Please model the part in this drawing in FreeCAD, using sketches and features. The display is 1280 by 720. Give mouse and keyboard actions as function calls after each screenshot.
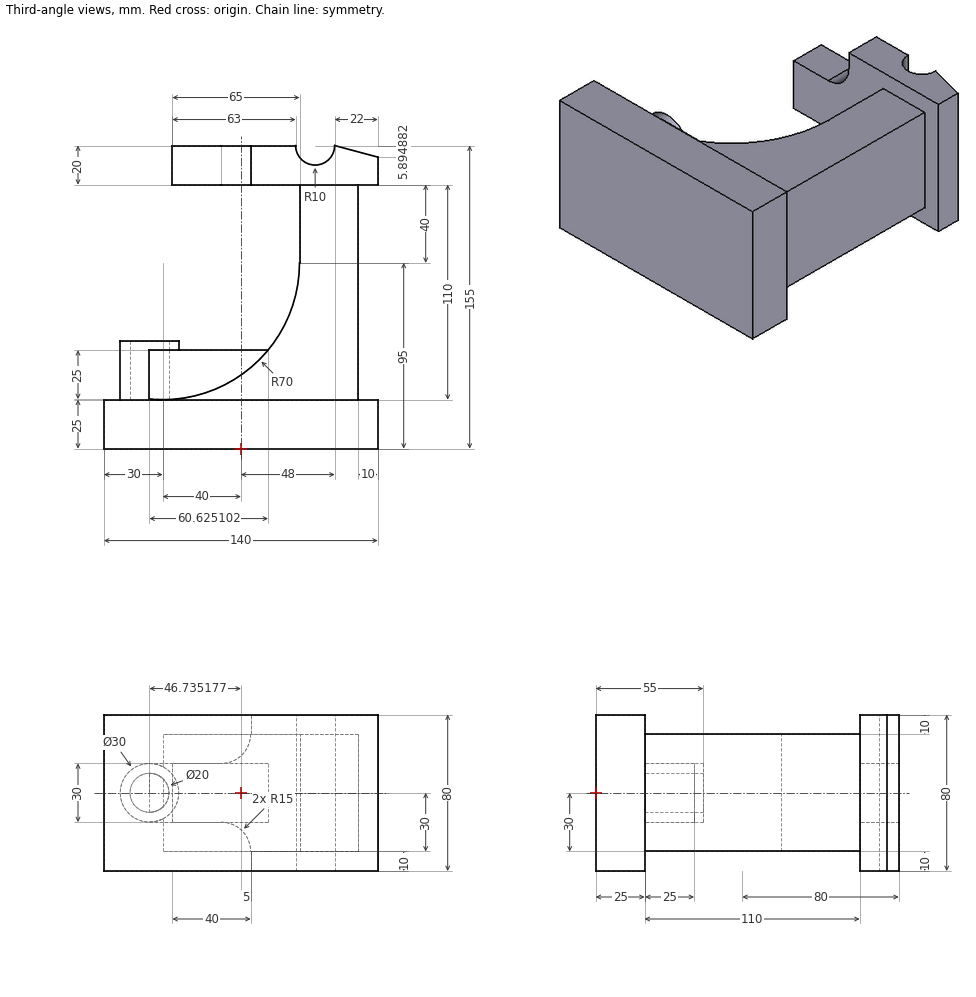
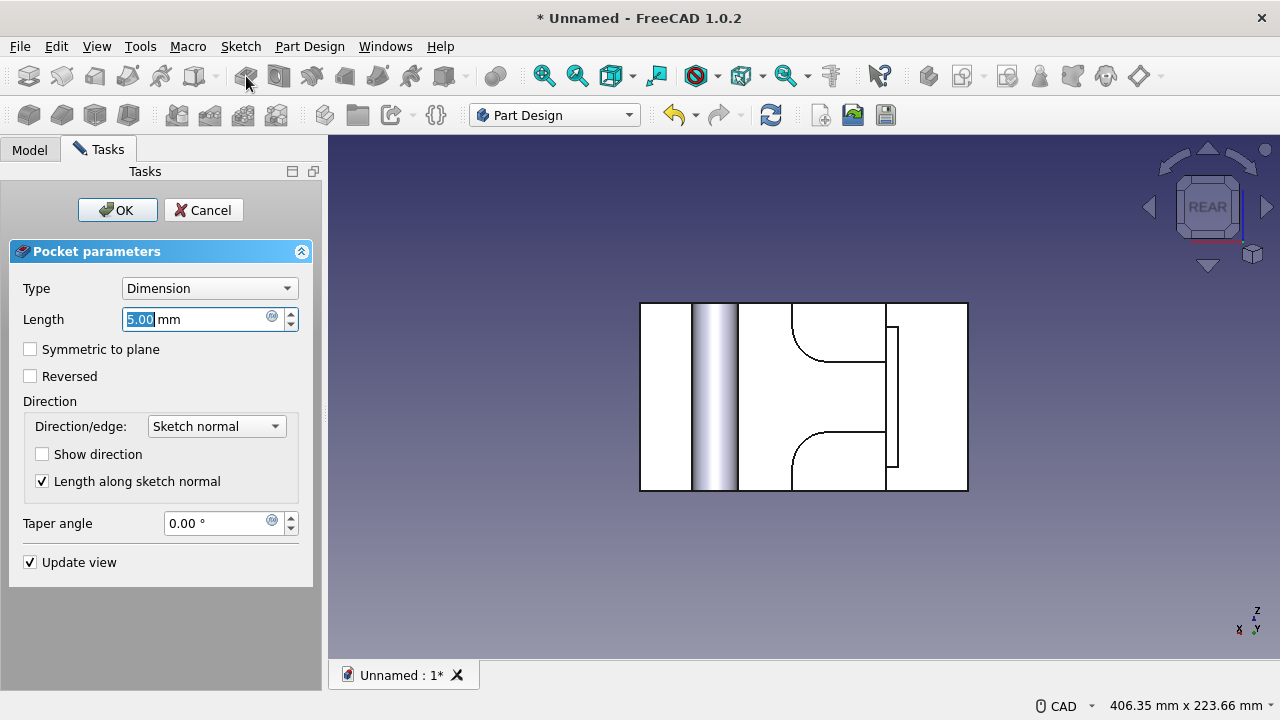
text(80)
key(Tab)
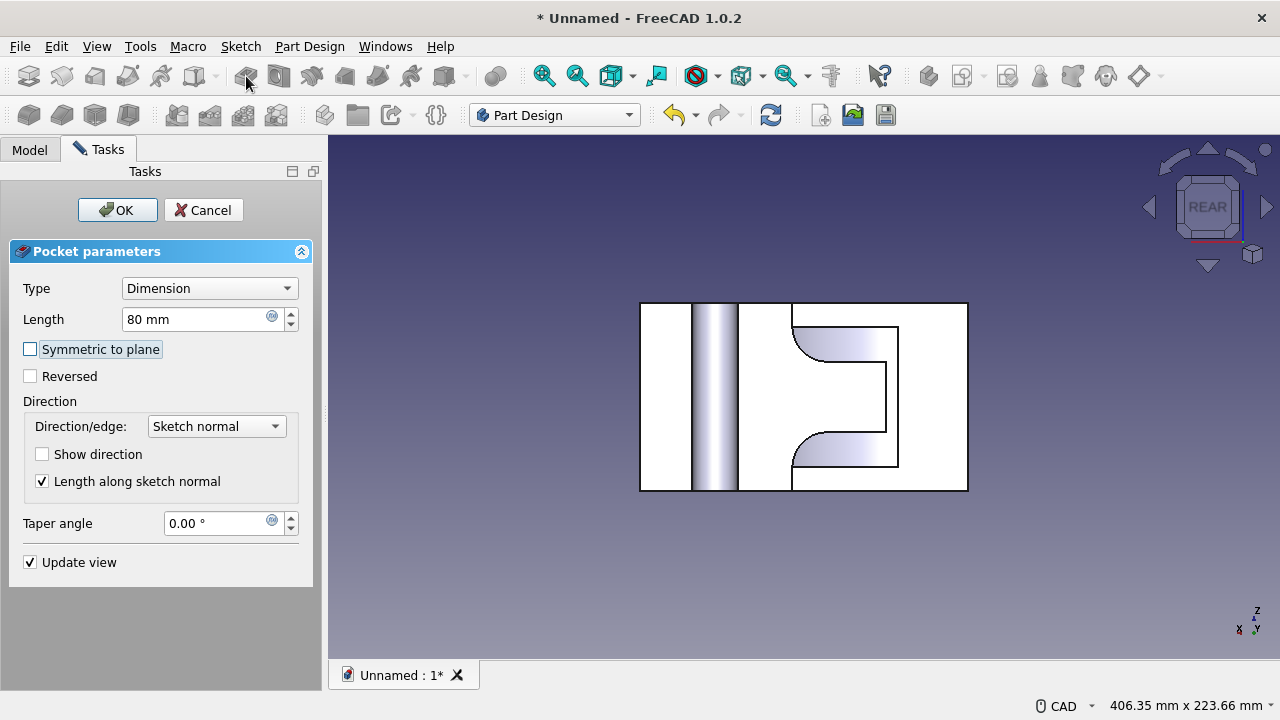
click(118, 210)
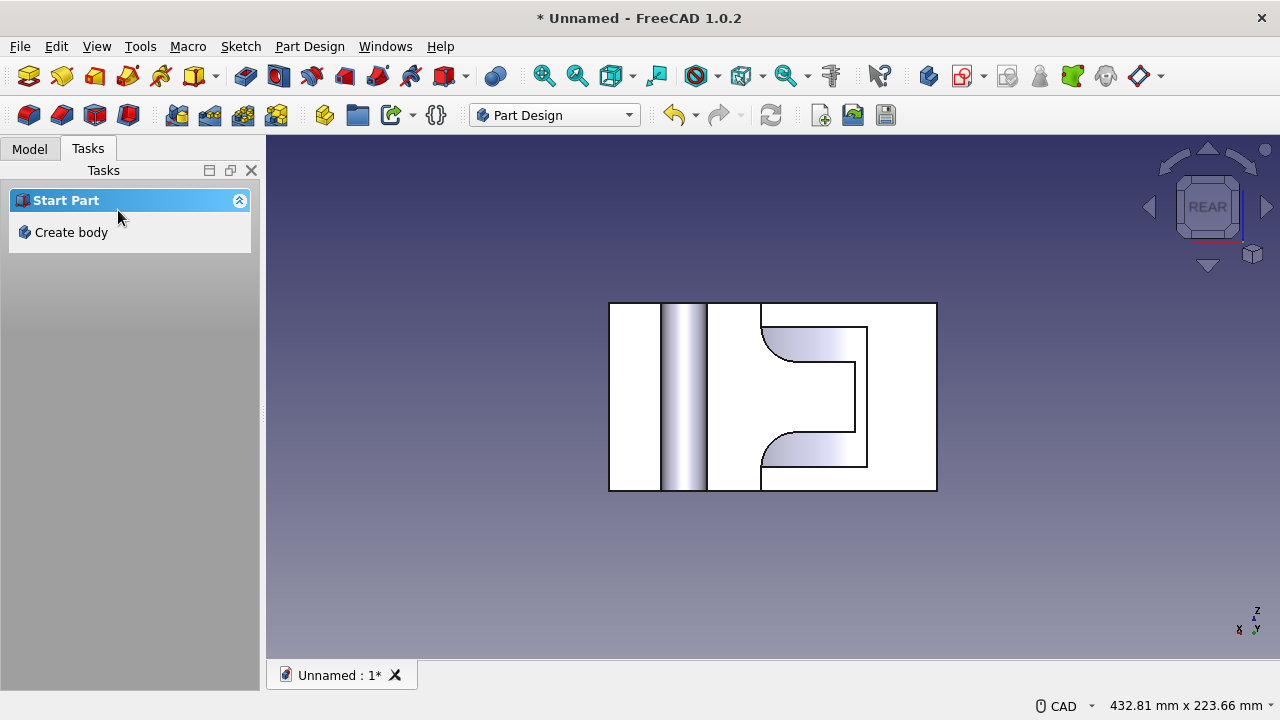
click(545, 76)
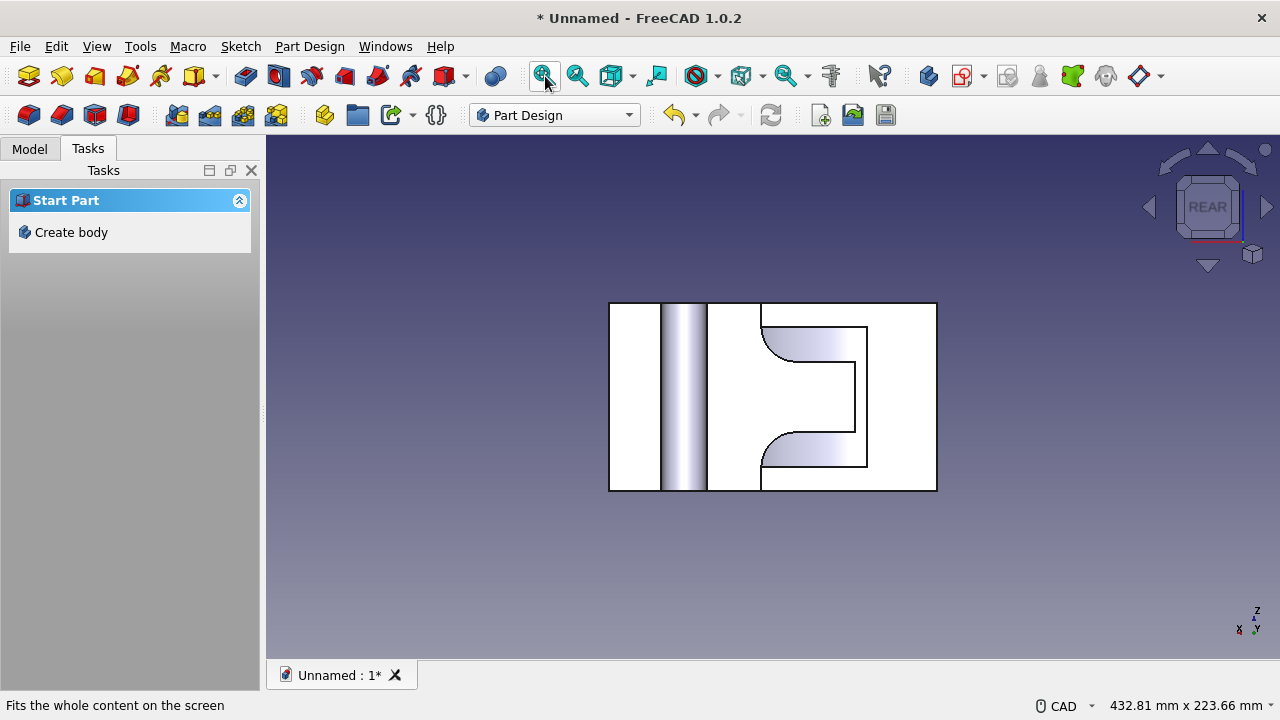
key(0)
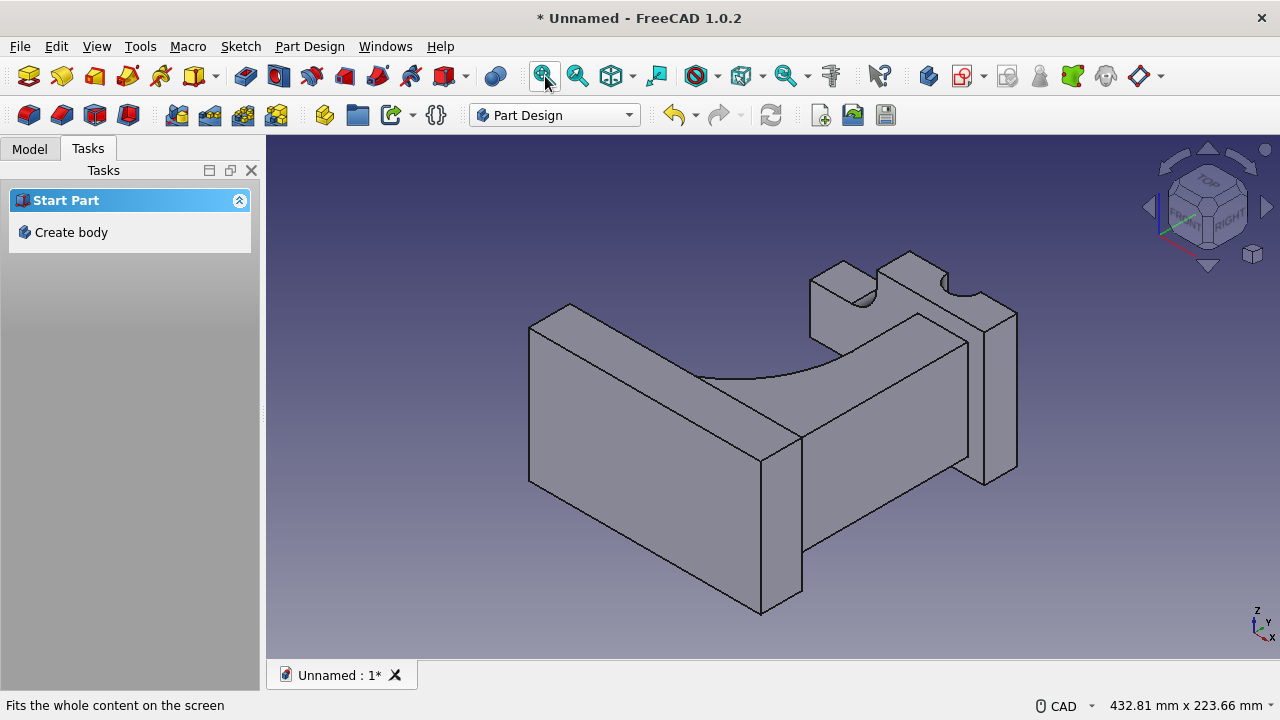
click(732, 420)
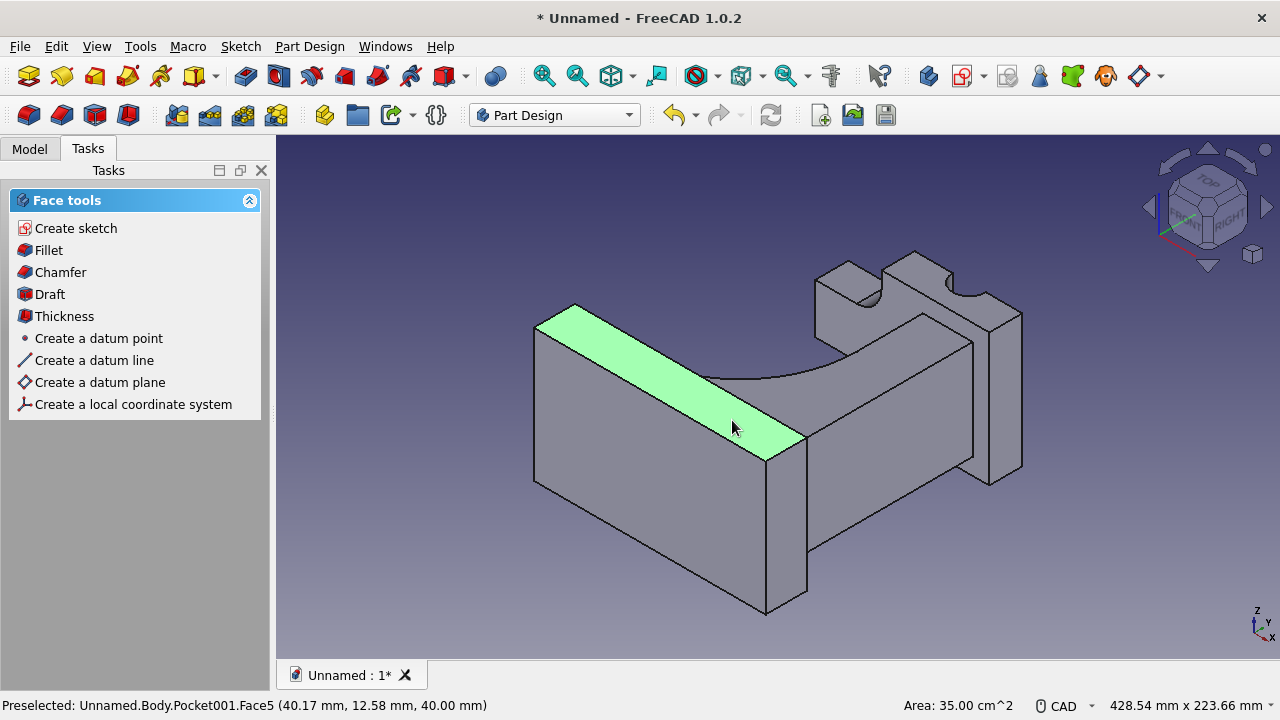
click(962, 76)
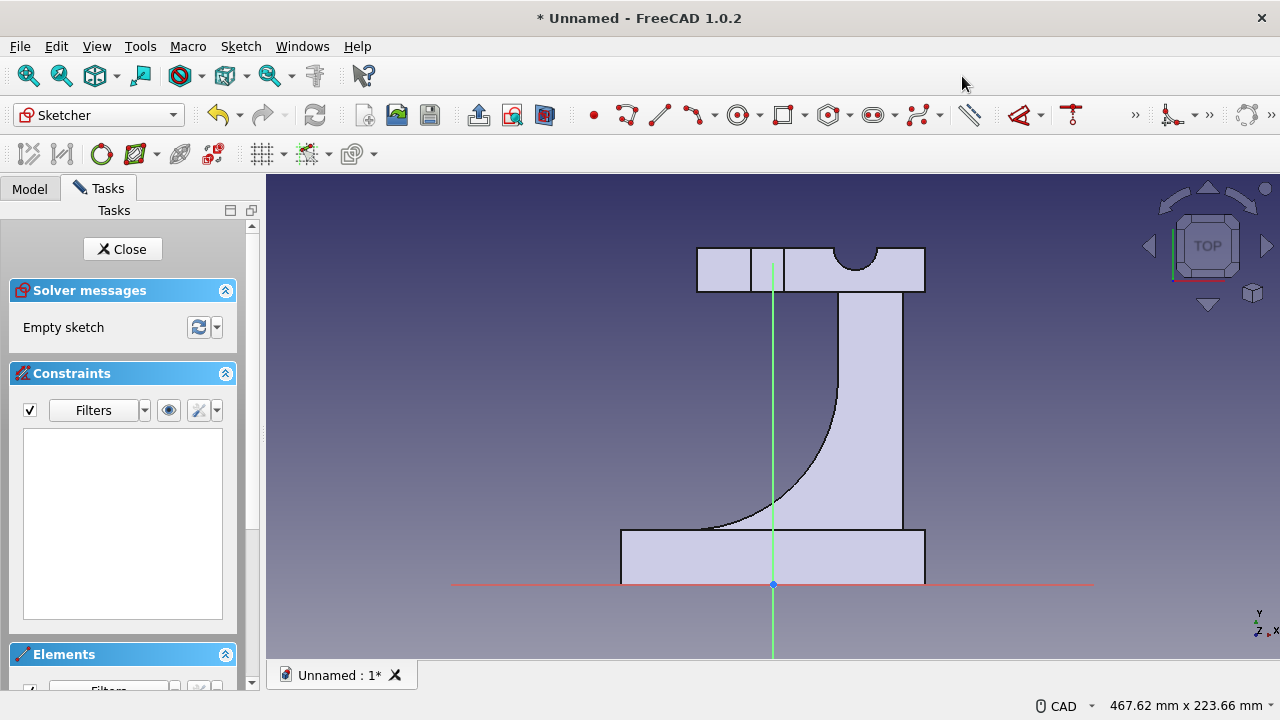
scroll(921, 239, up, 12)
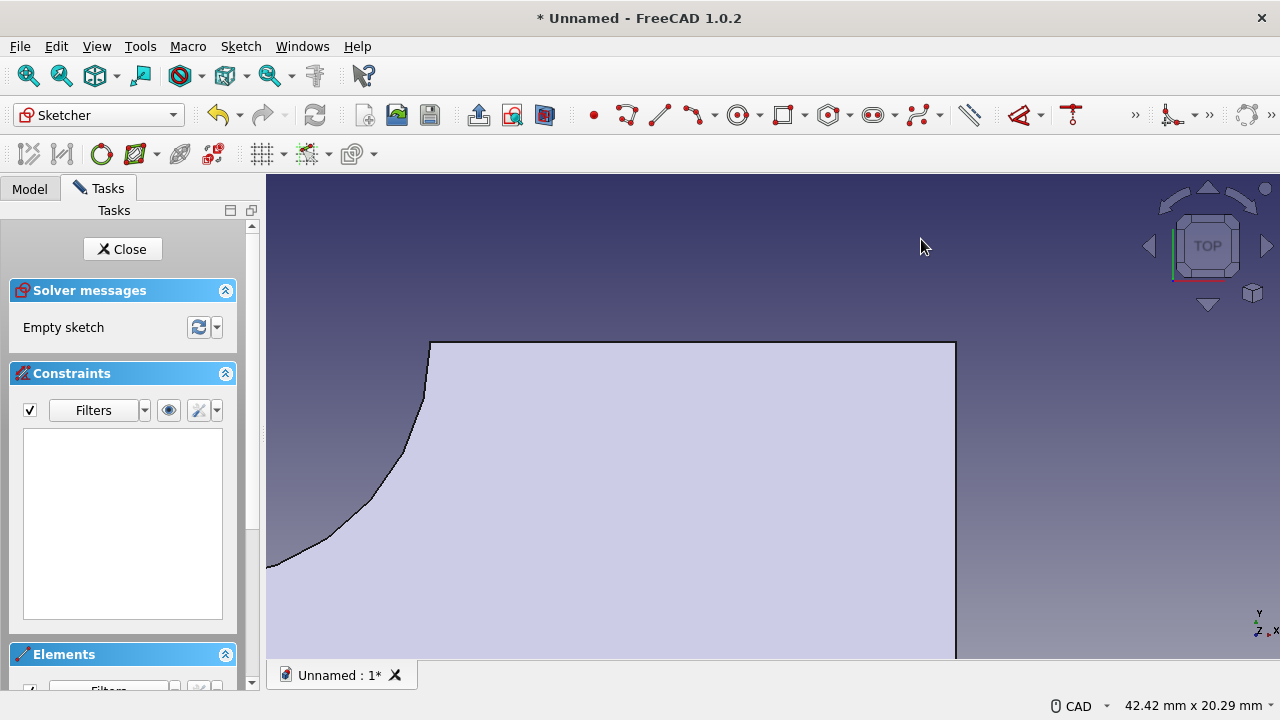
click(627, 116)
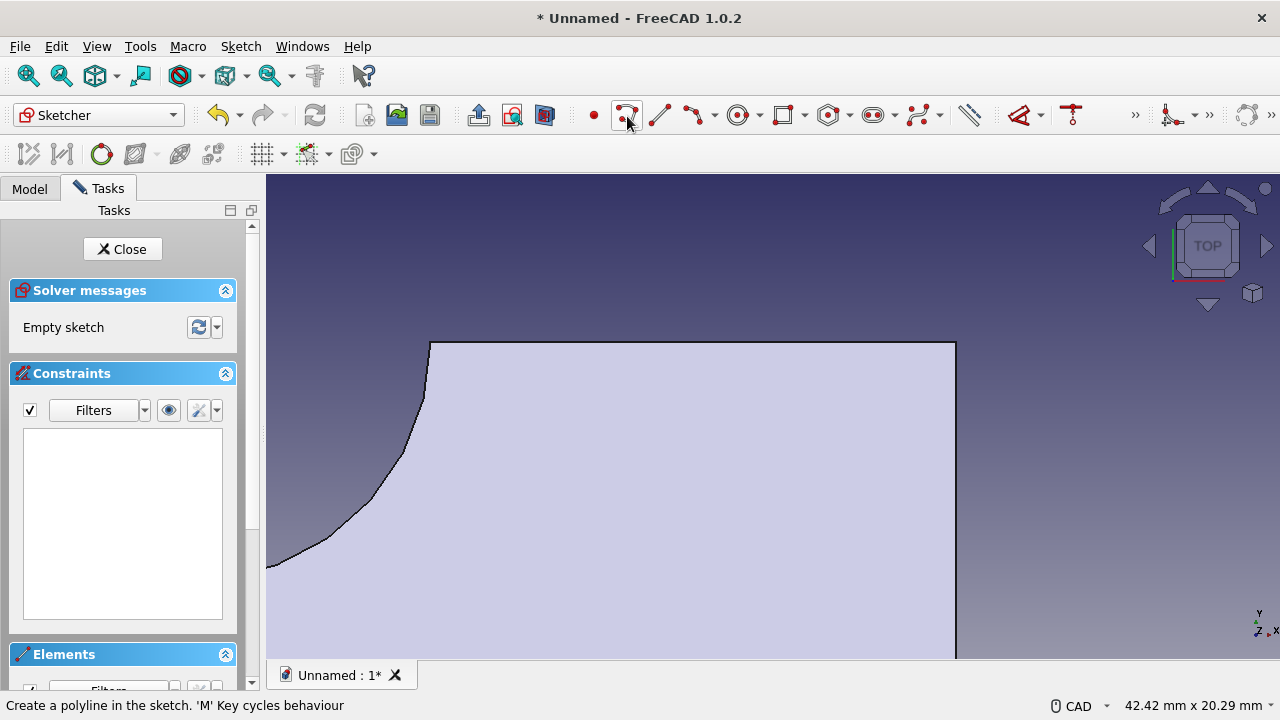
click(430, 342)
click(956, 483)
click(956, 342)
click(430, 343)
key(Escape)
key(Escape)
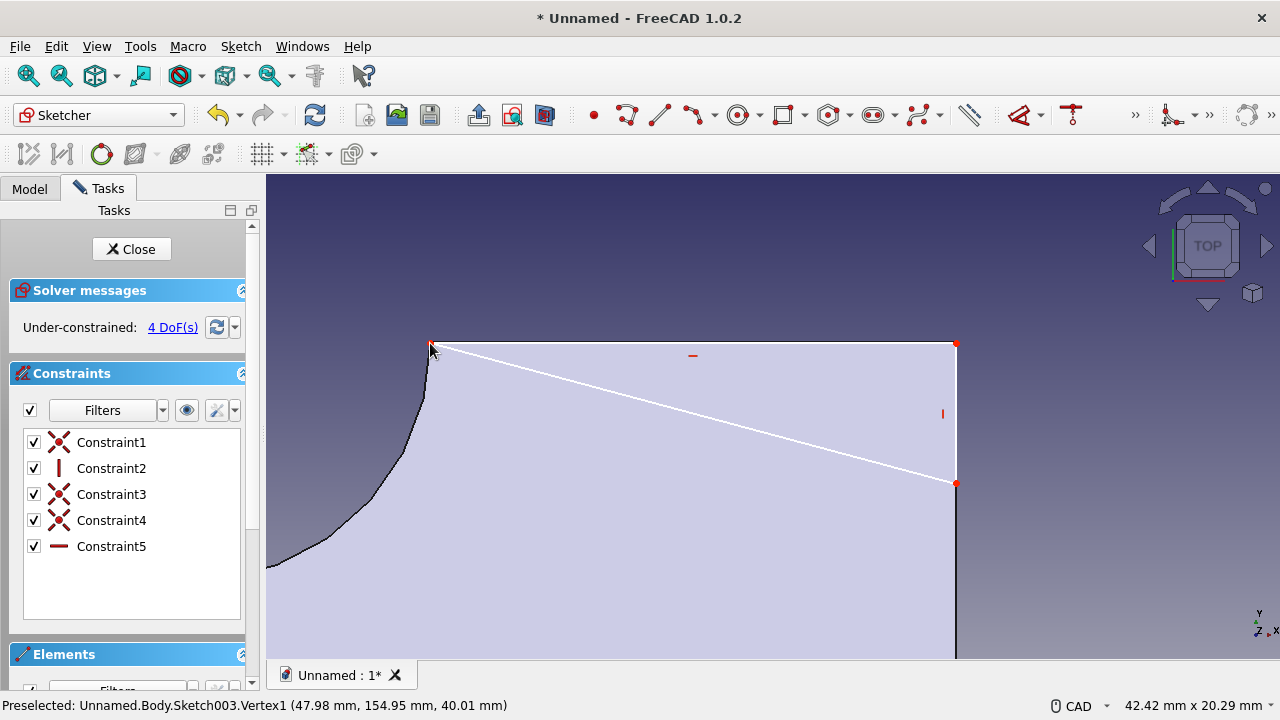
click(1018, 116)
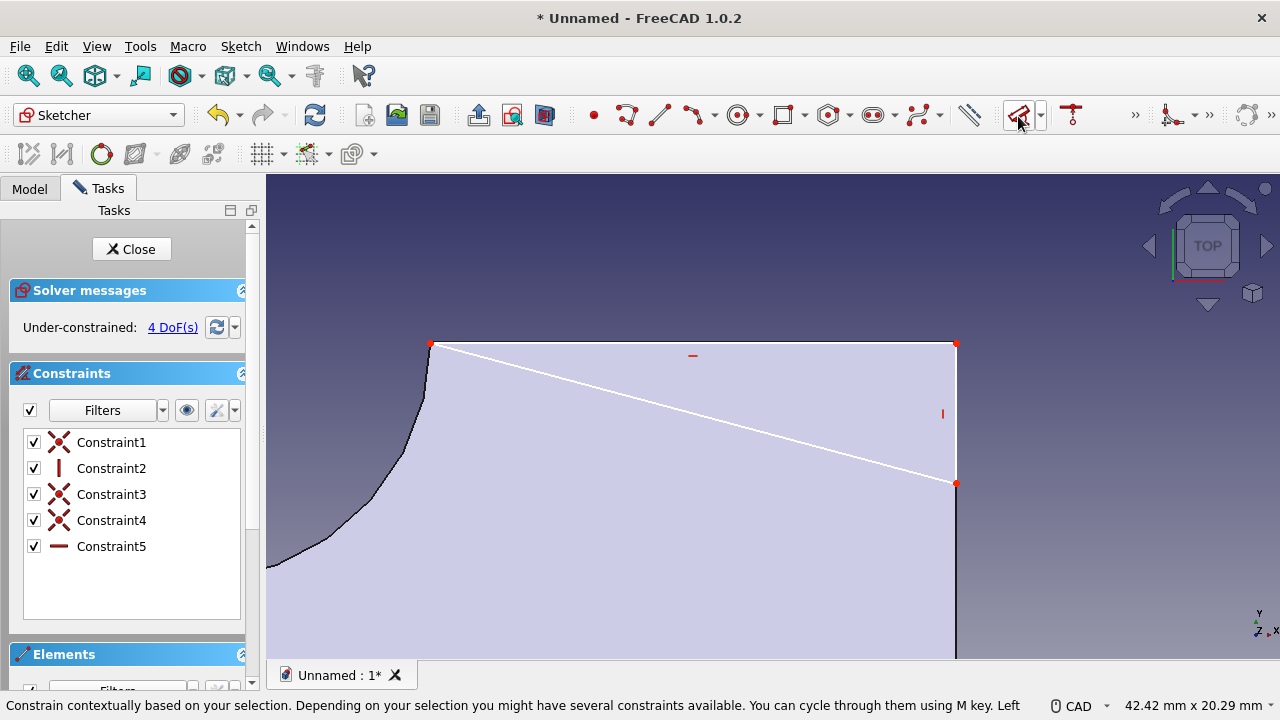
click(798, 343)
click(693, 309)